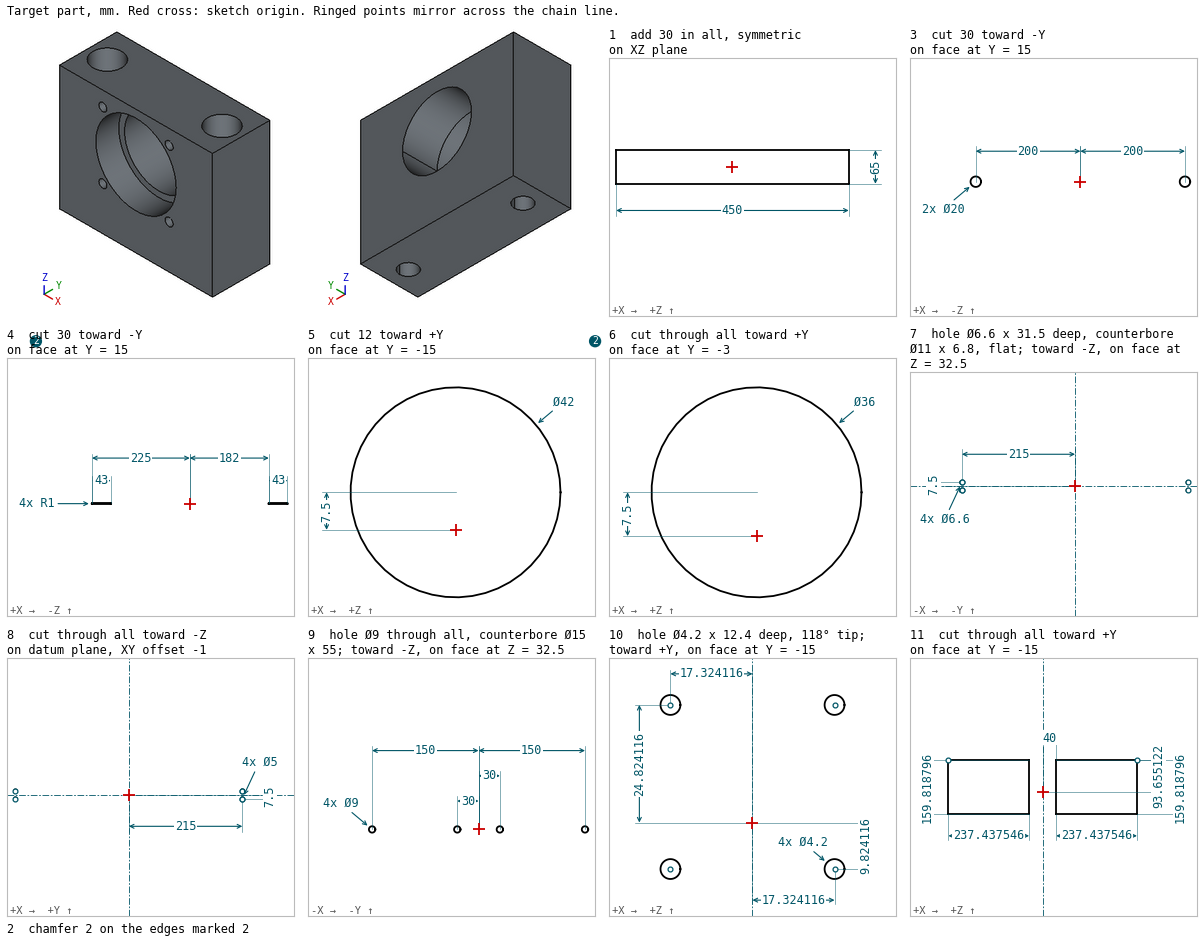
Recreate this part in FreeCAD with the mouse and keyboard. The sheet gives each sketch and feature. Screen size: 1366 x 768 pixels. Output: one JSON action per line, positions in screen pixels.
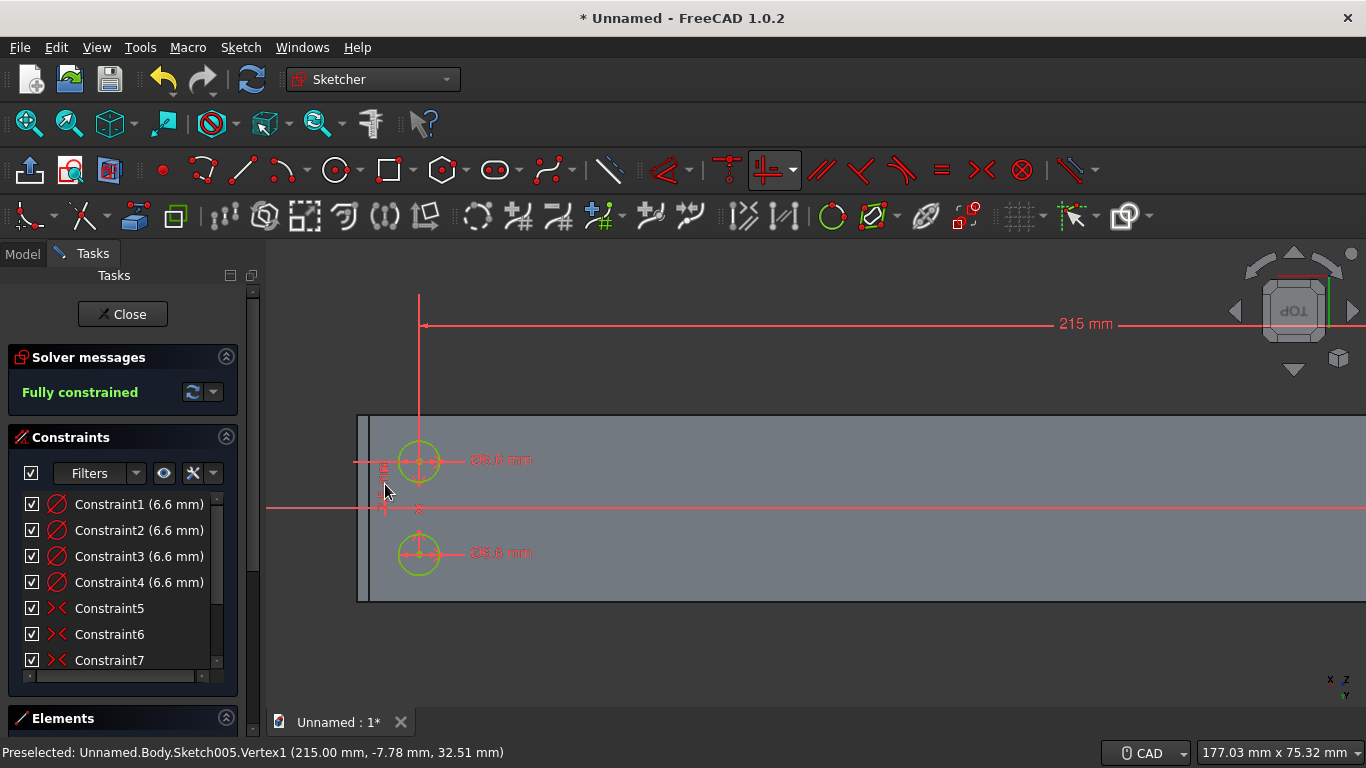
{"action": "left_click", "coordinate": [123, 314]}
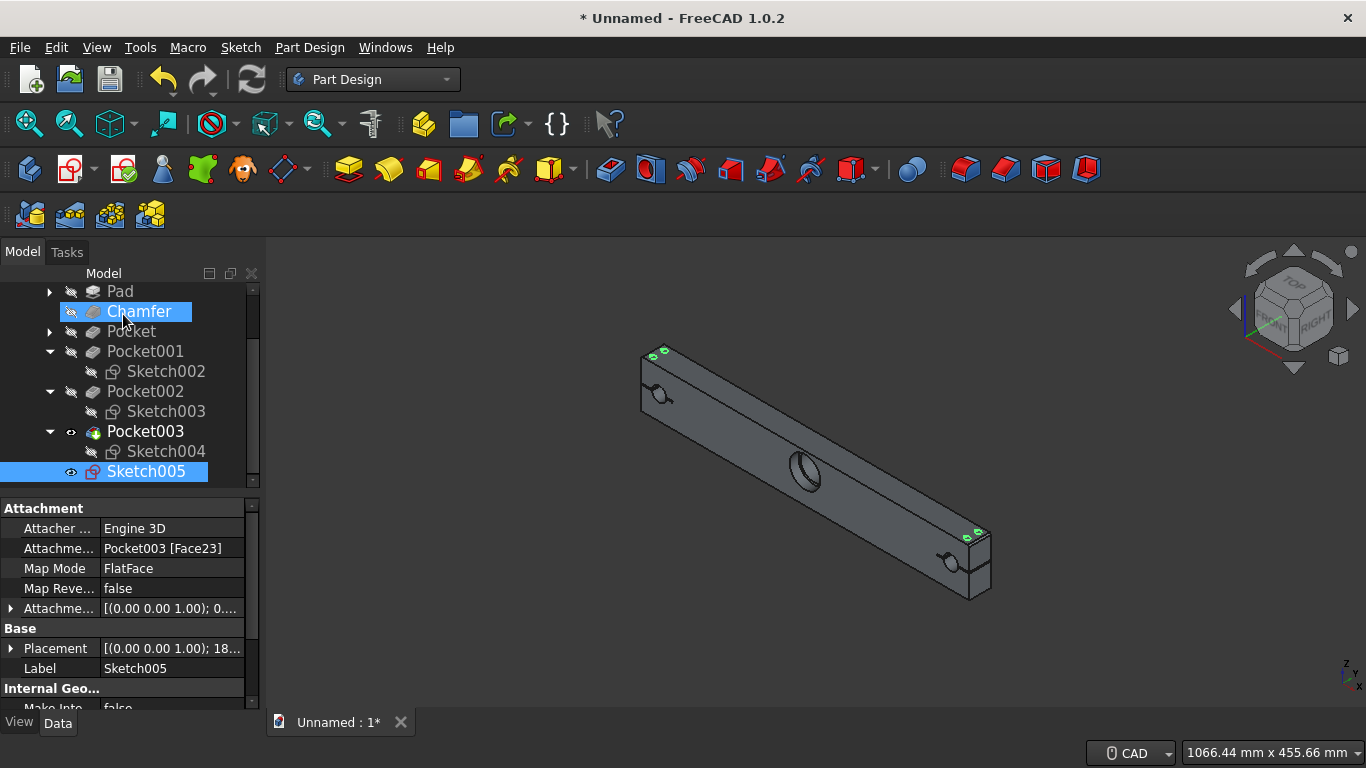
{"action": "left_click", "coordinate": [652, 170]}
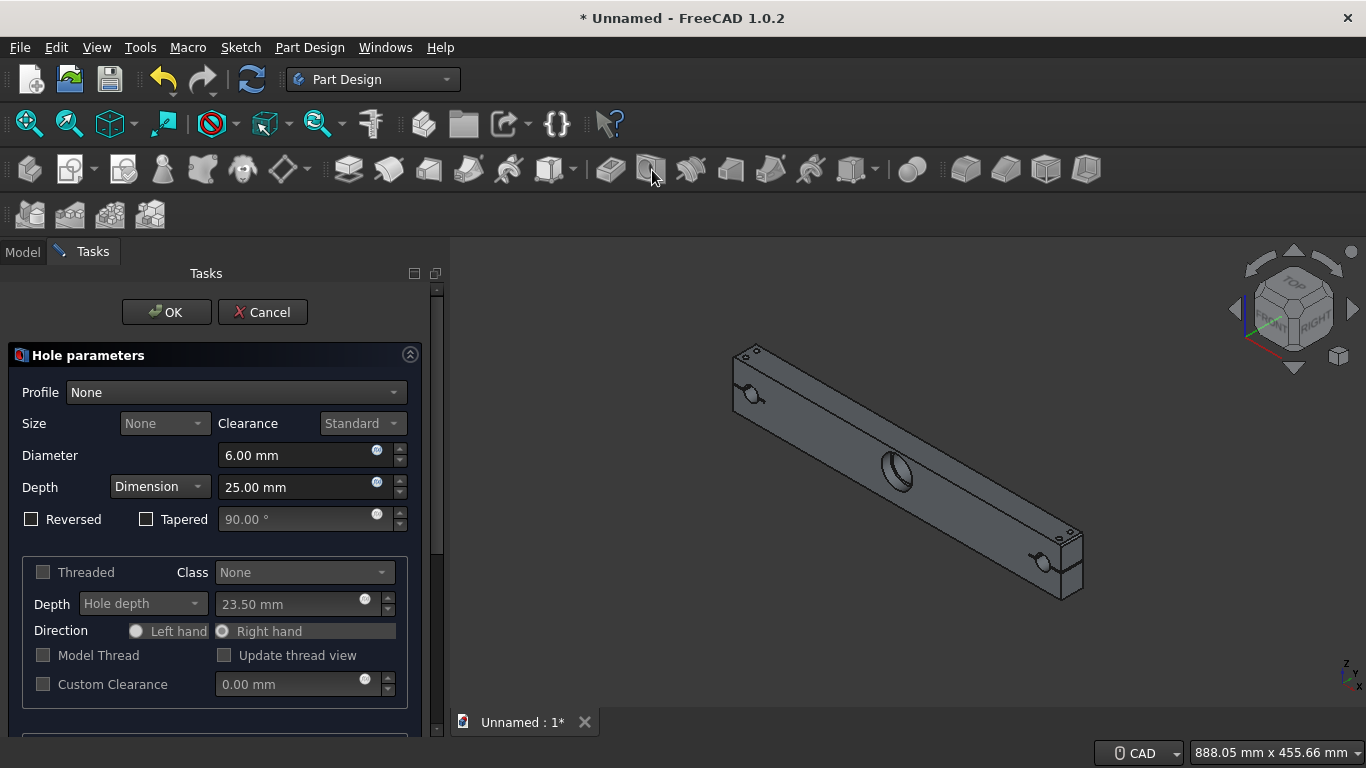
{"action": "triple_click", "coordinate": [305, 455]}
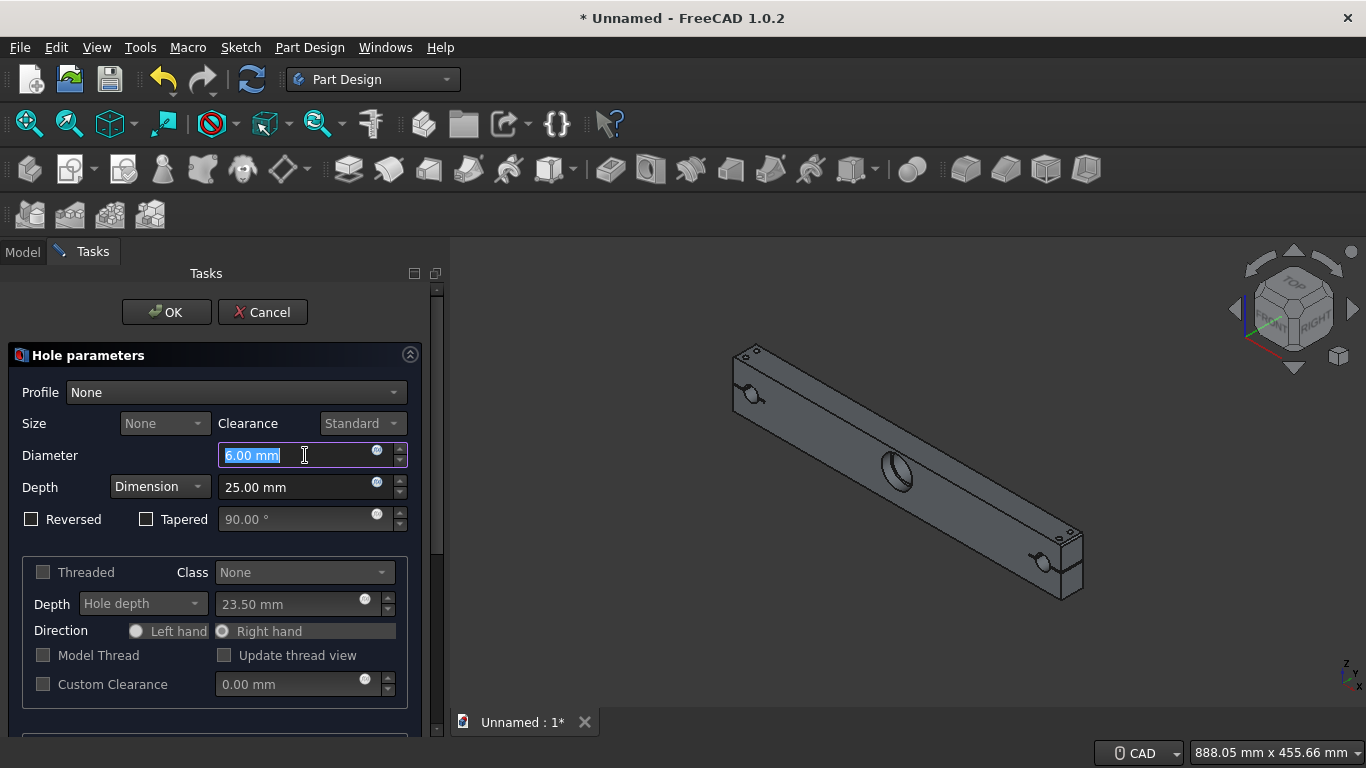
{"action": "type", "text": "6.6"}
{"action": "key", "text": "Tab"}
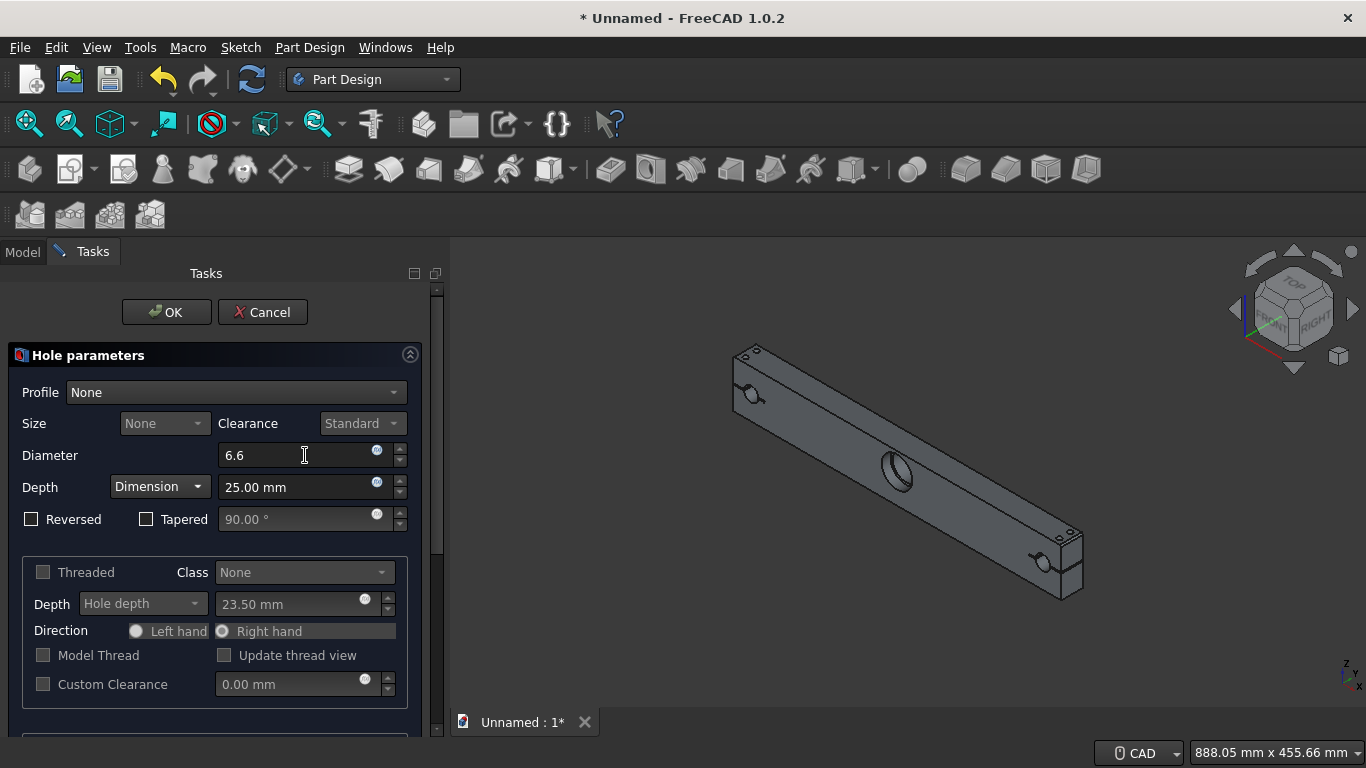
{"action": "triple_click", "coordinate": [305, 487]}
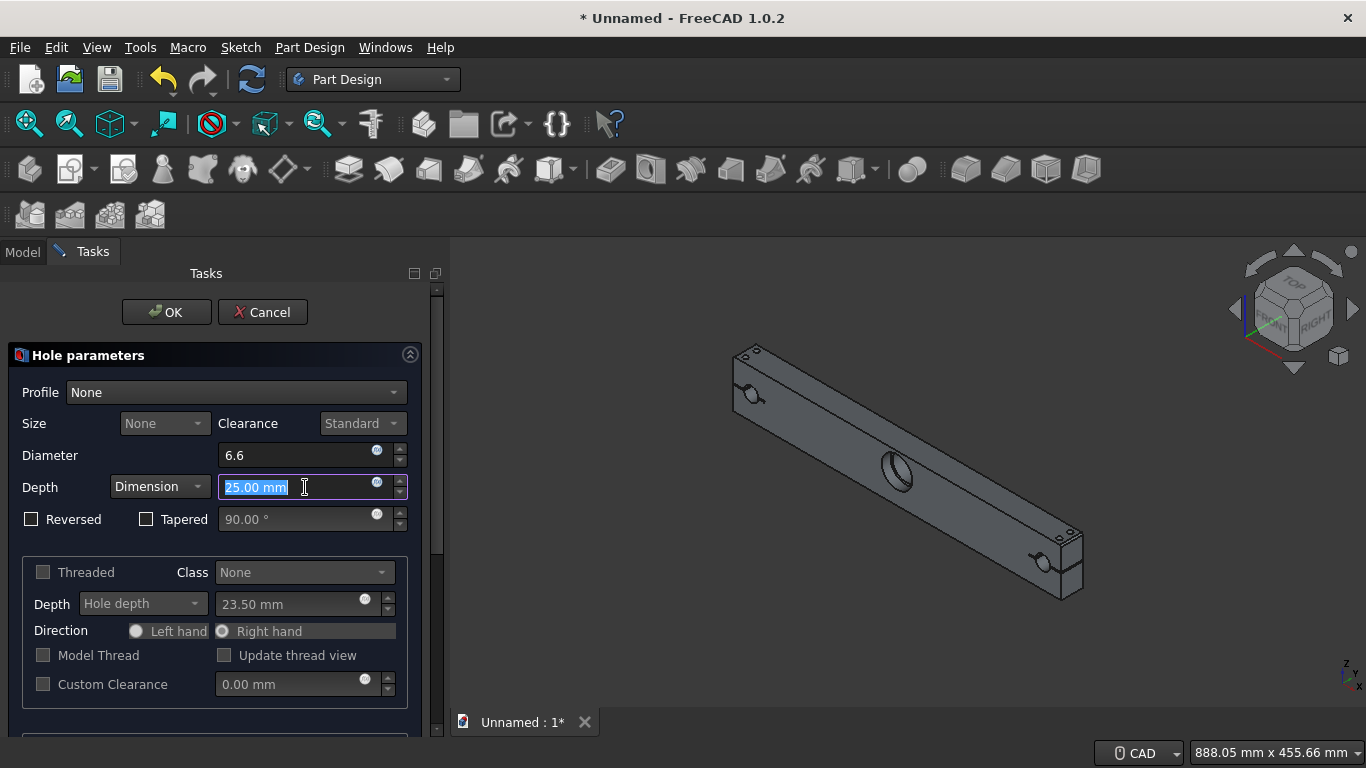
{"action": "type", "text": "31.5"}
{"action": "key", "text": "Tab"}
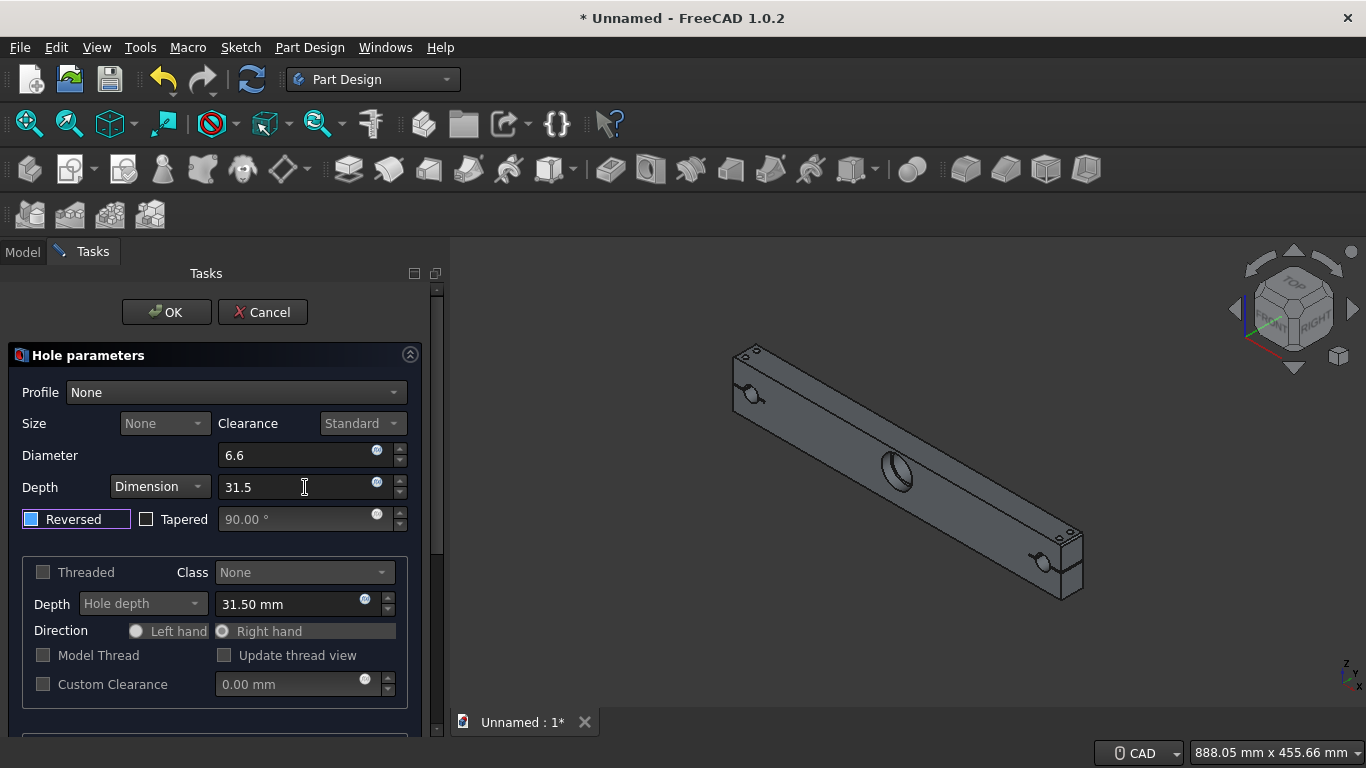
{"action": "scroll", "coordinate": [437, 510], "scroll_direction": "down", "scroll_amount": 2}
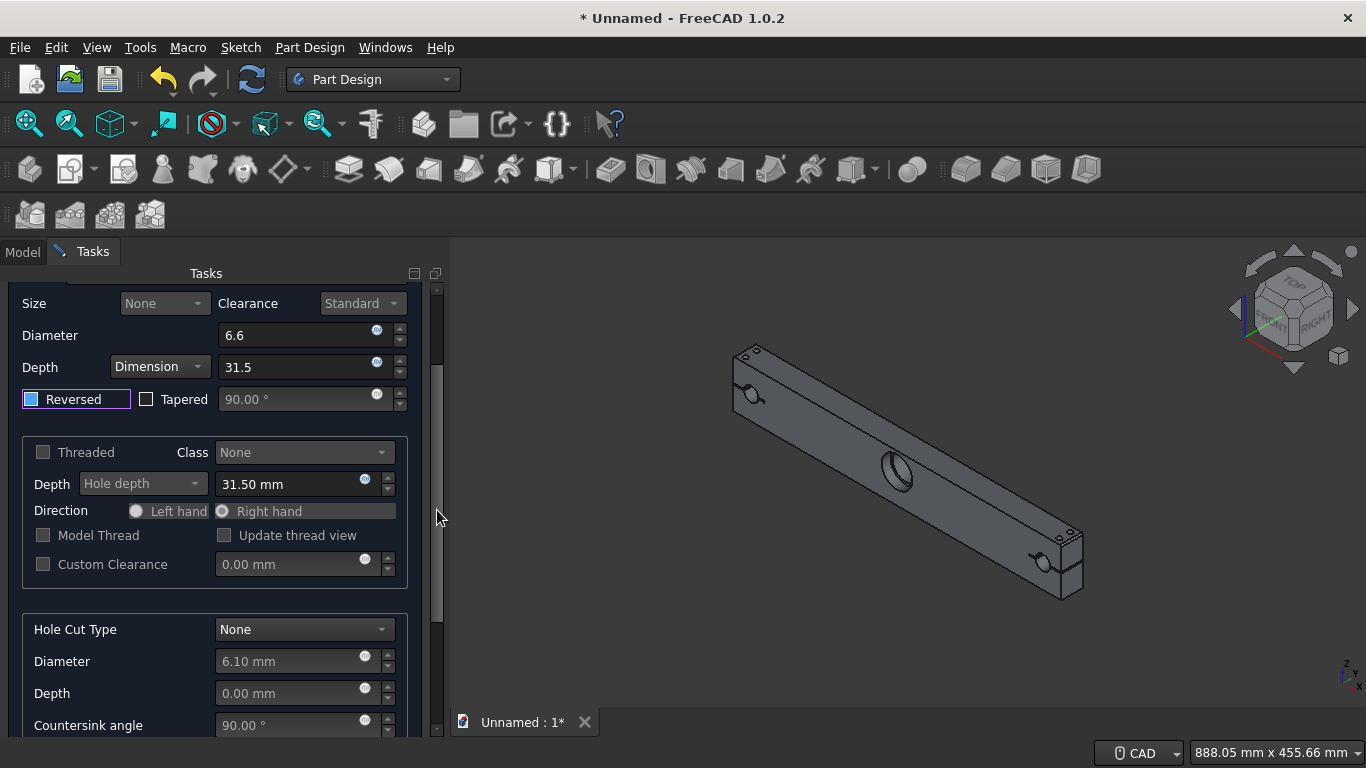
{"action": "left_click", "coordinate": [306, 630]}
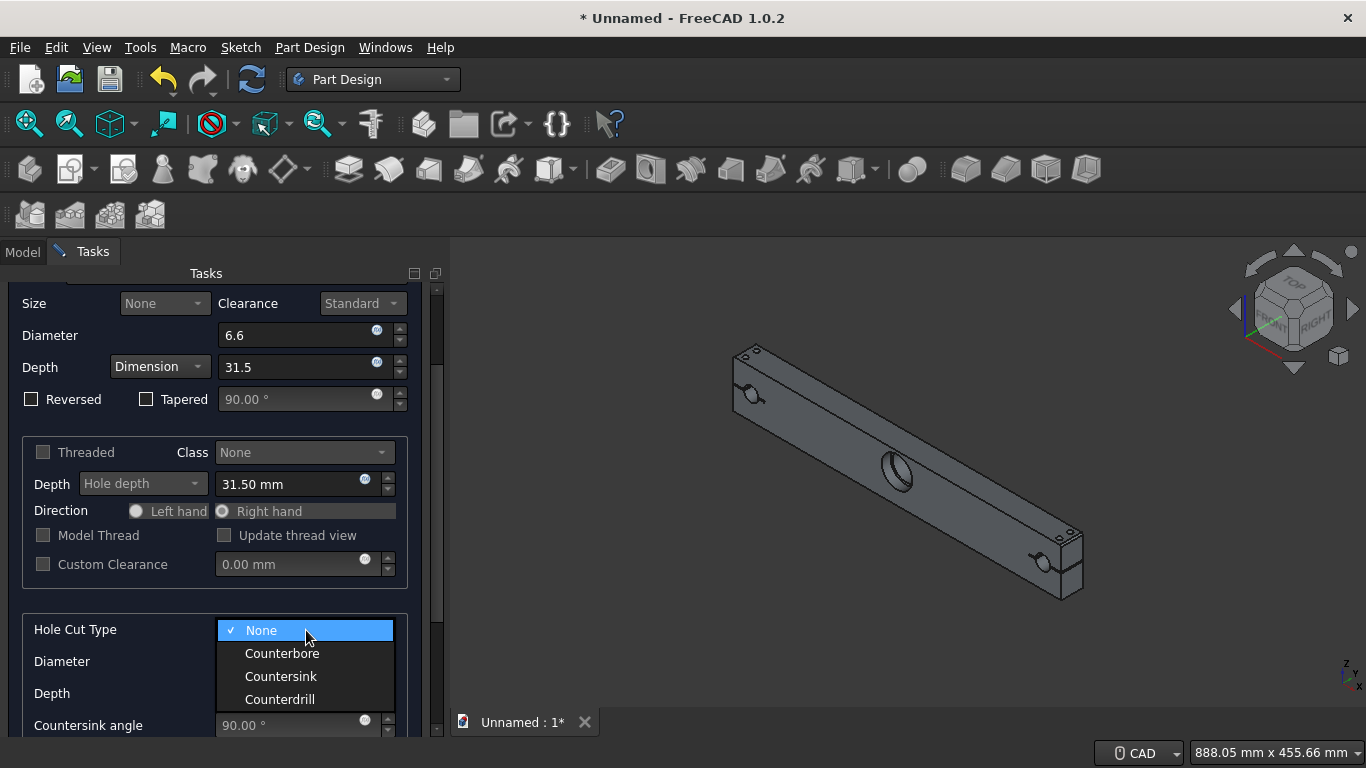
{"action": "left_click", "coordinate": [304, 654]}